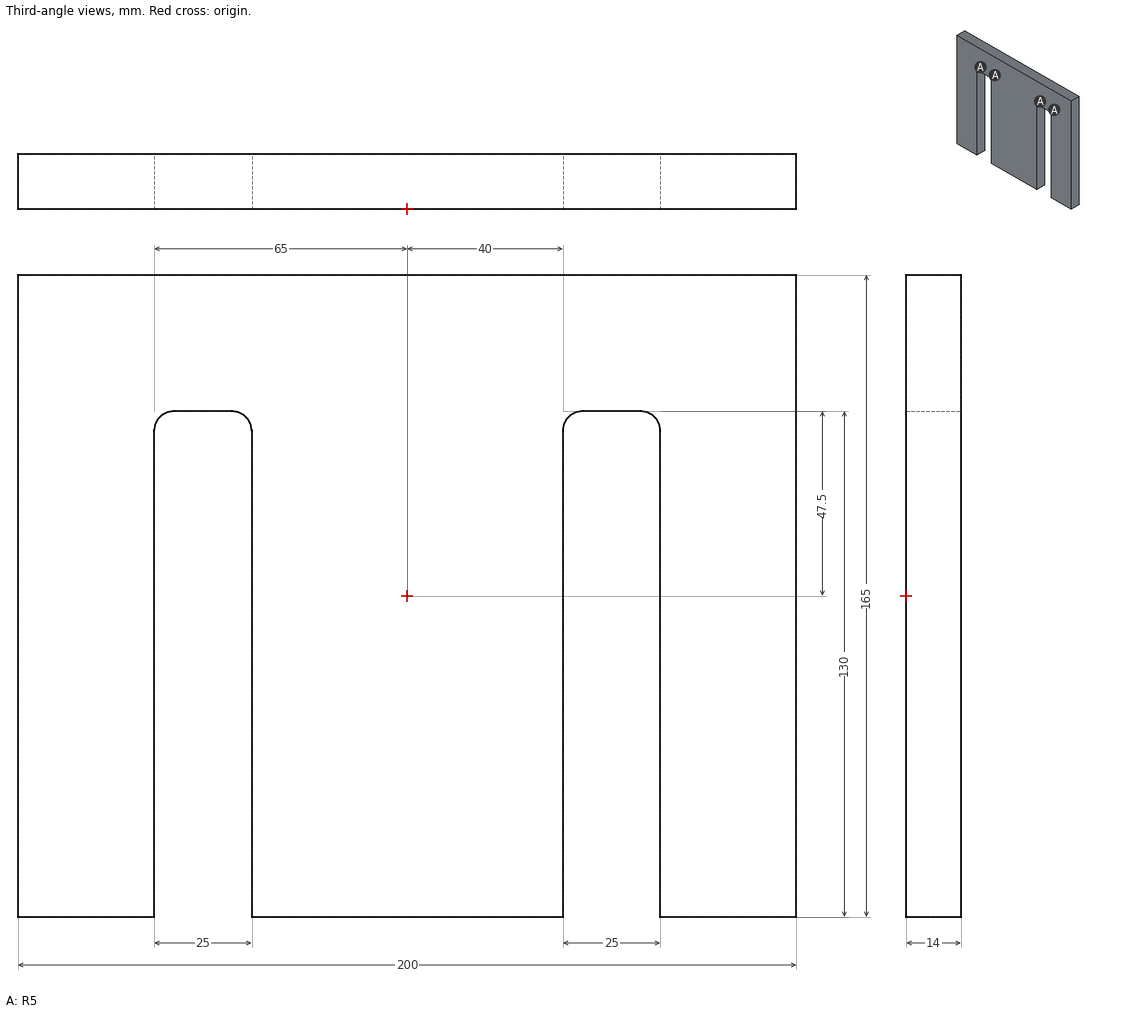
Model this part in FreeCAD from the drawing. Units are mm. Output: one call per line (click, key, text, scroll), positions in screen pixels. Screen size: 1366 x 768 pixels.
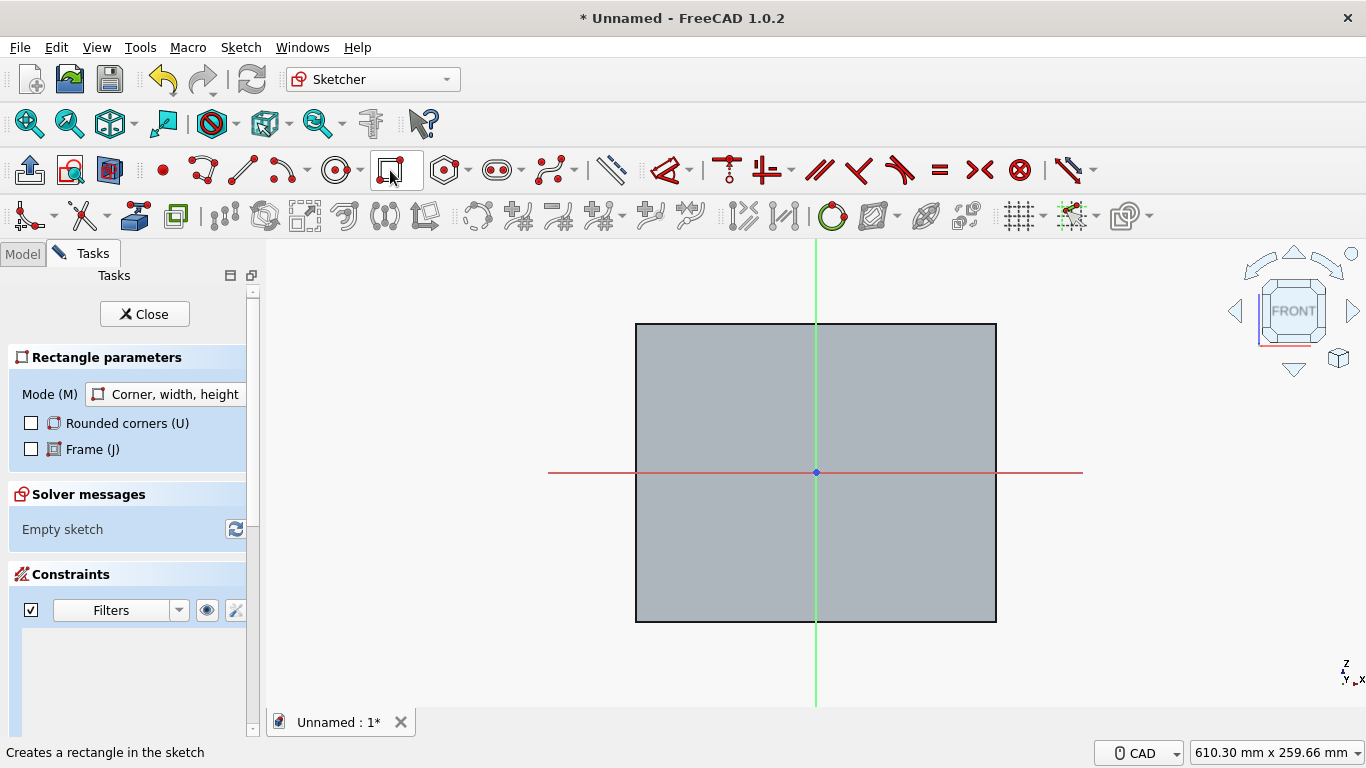
click(888, 387)
move(933, 622)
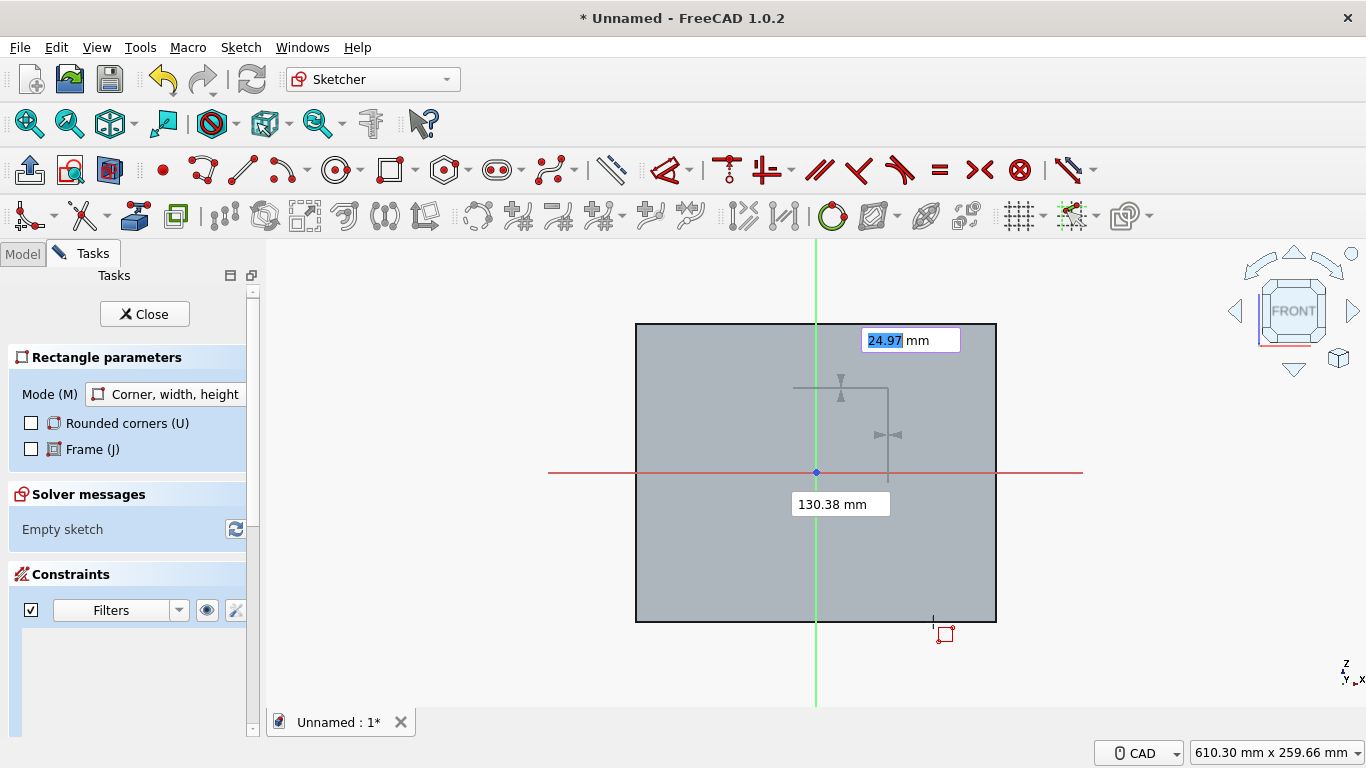
text(25)
key(Tab)
text(130)
key(Return)
key(Escape)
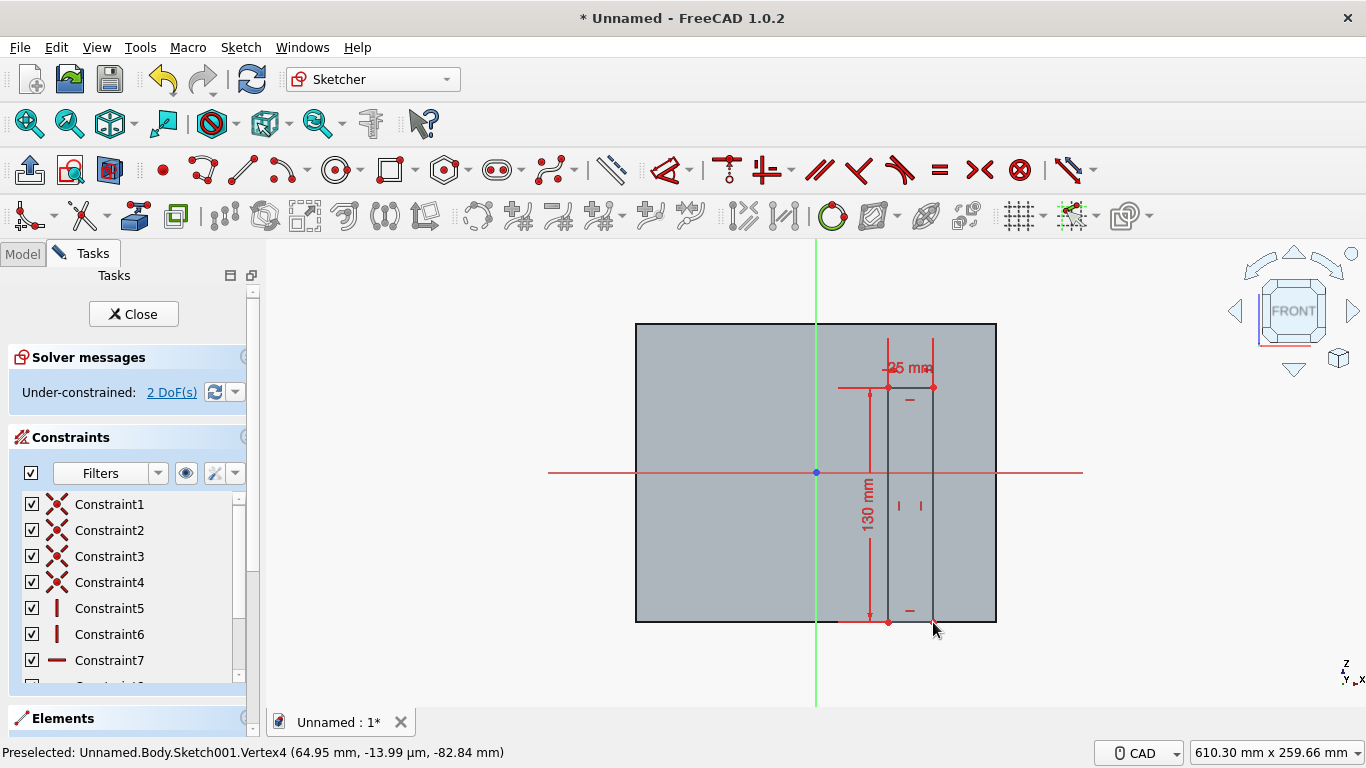
click(666, 170)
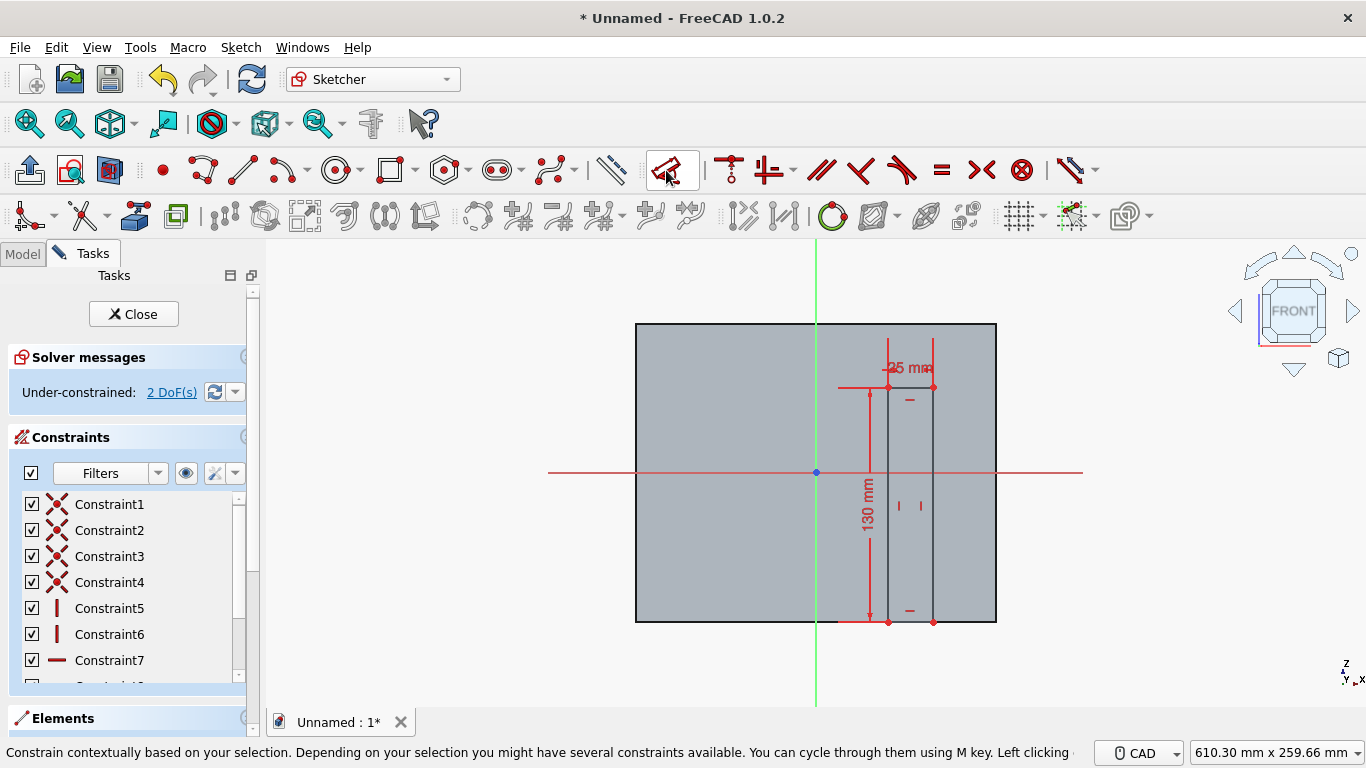
click(888, 388)
click(852, 354)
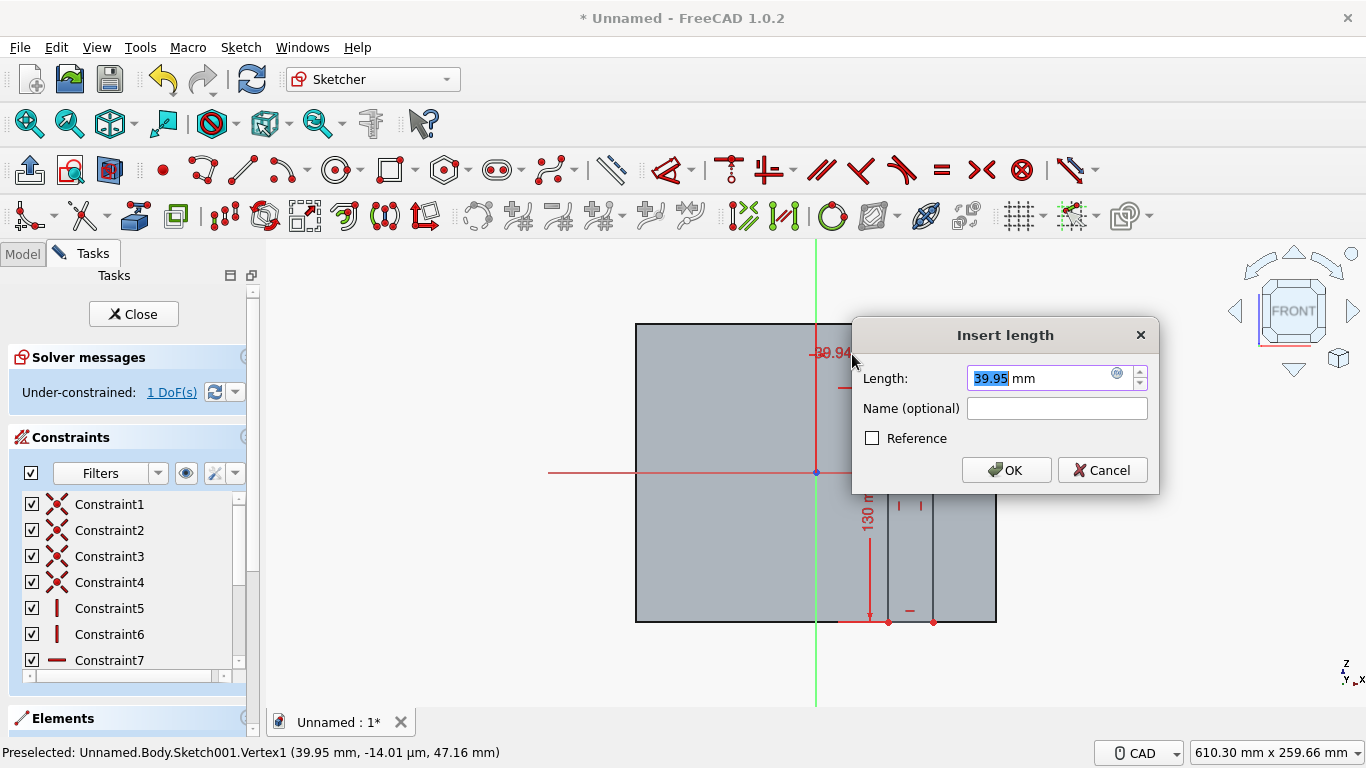
text(40)
key(Return)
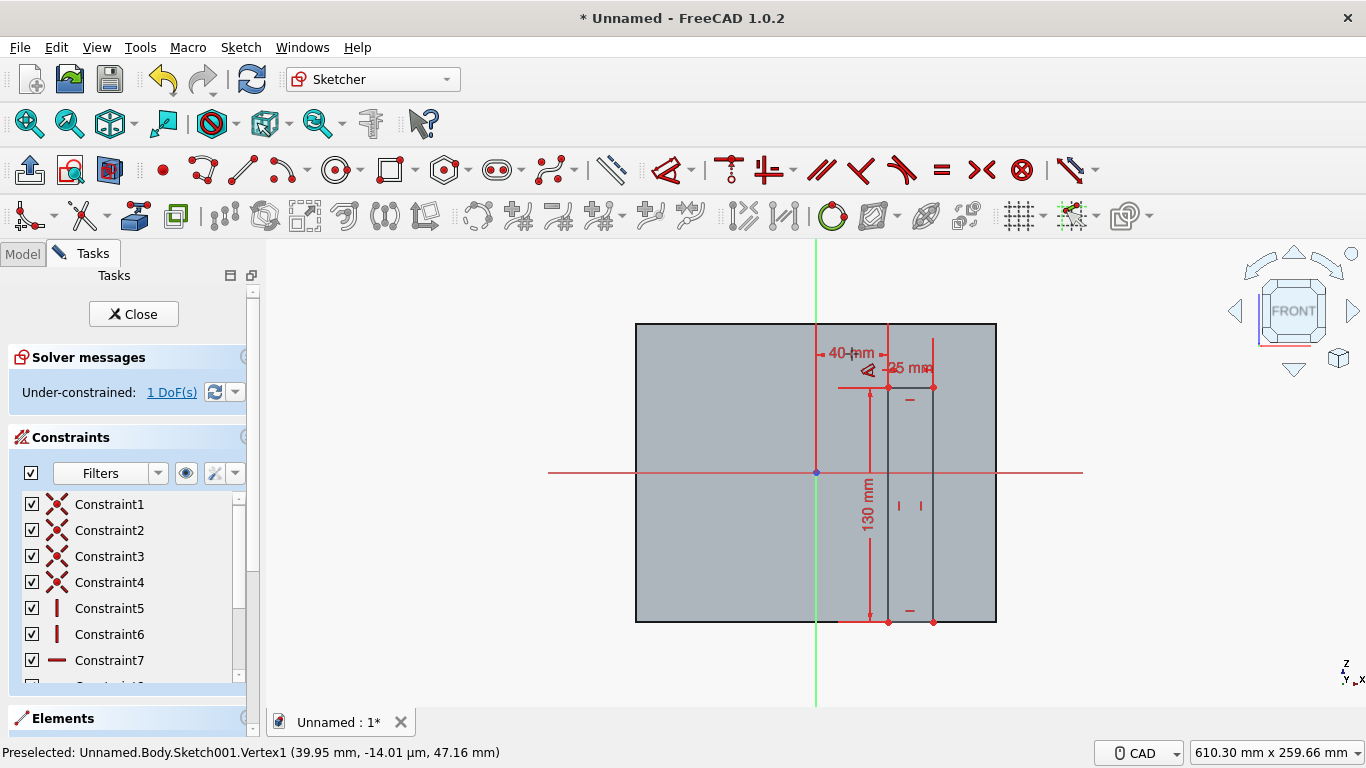
click(888, 388)
click(782, 430)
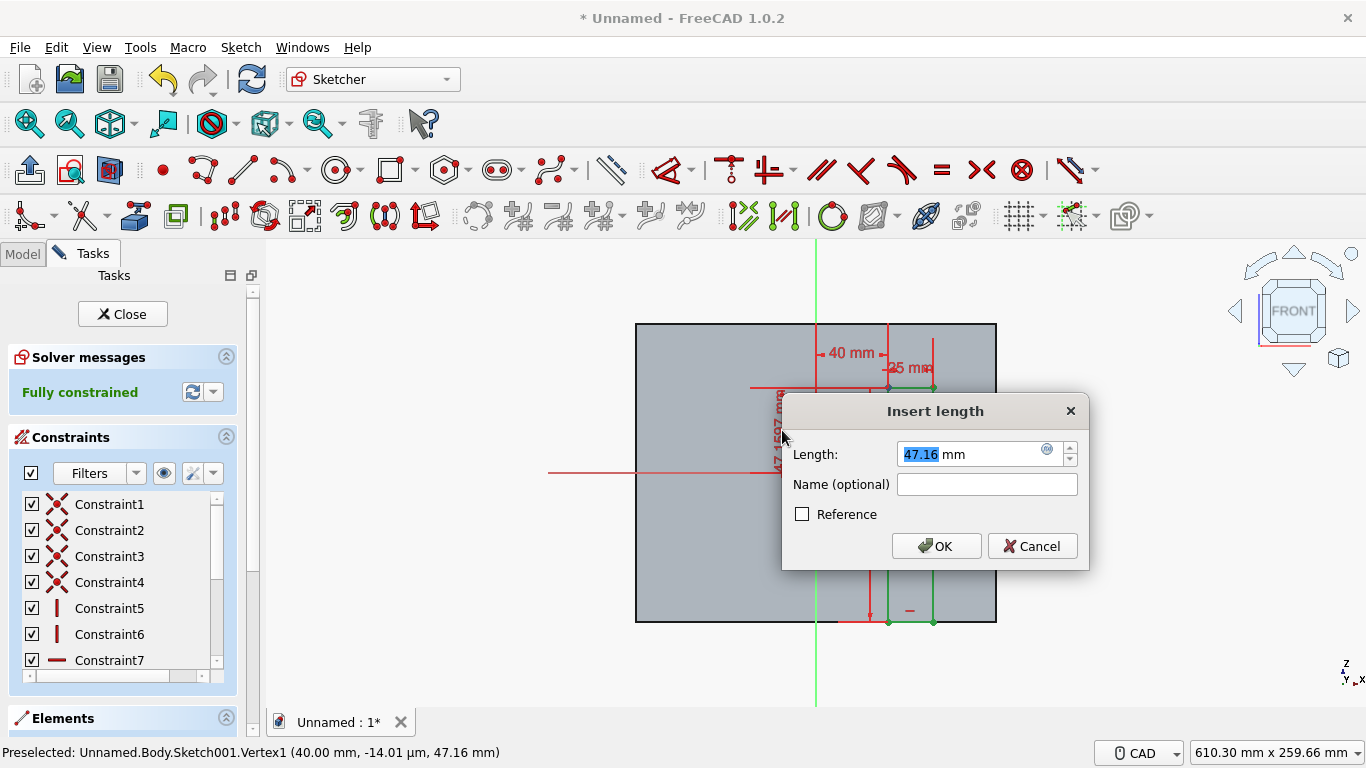
text(47.5)
key(Return)
key(Escape)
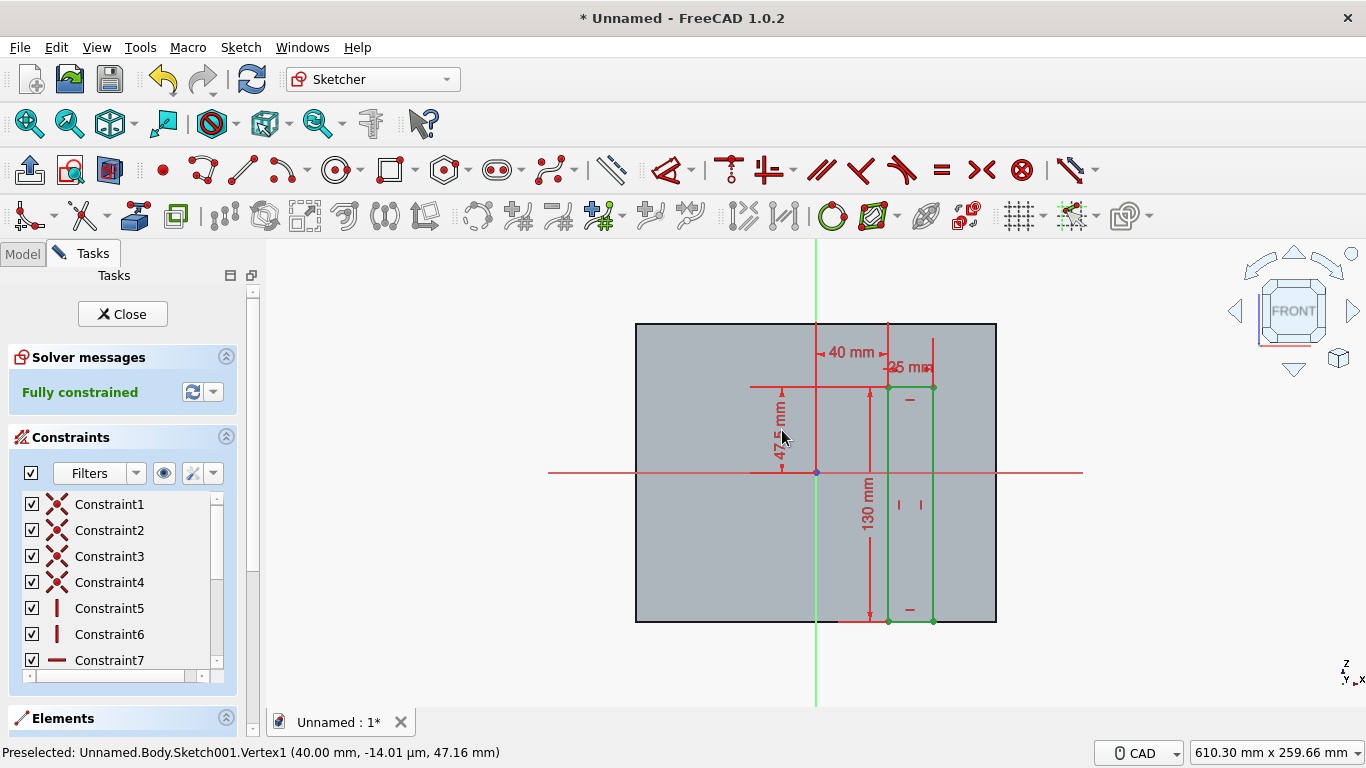
click(123, 314)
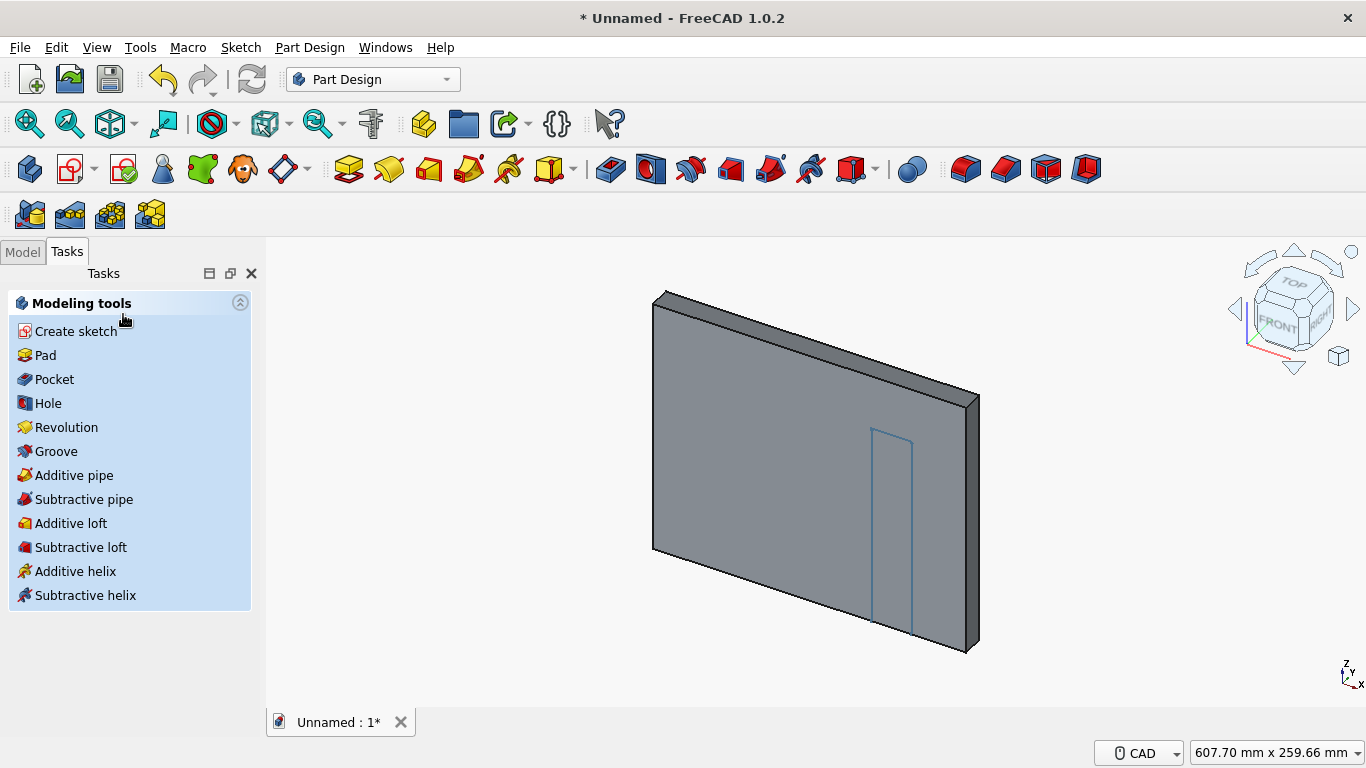
click(612, 170)